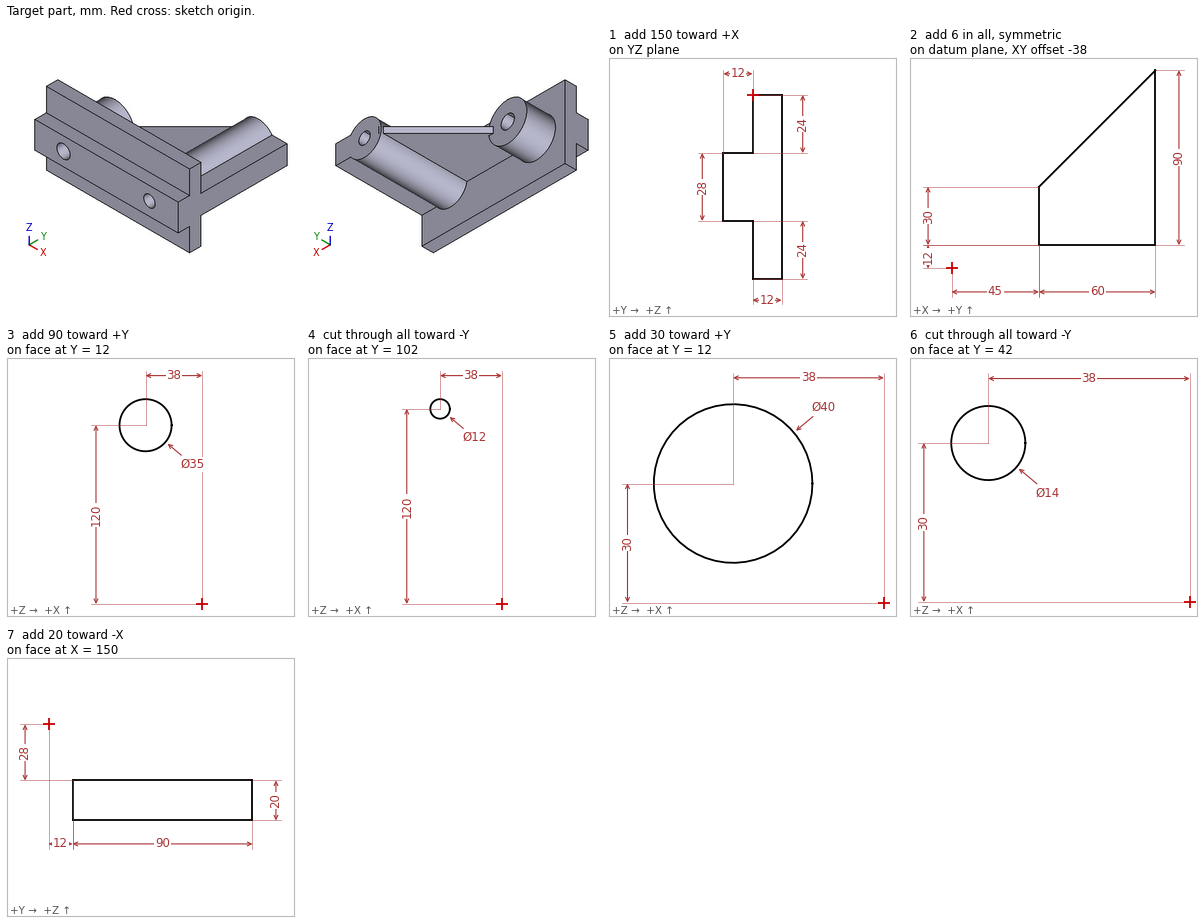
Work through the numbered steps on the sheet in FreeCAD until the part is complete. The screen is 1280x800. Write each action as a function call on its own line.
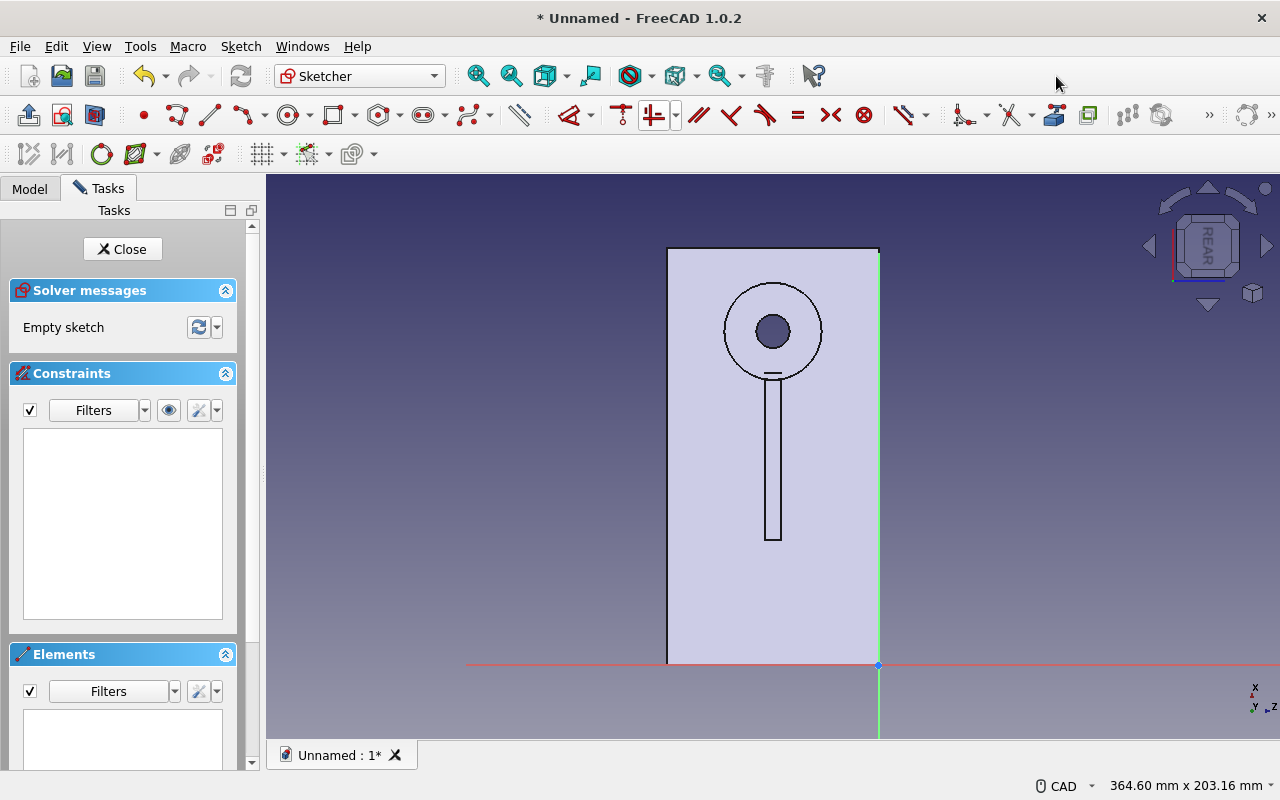
click(95, 116)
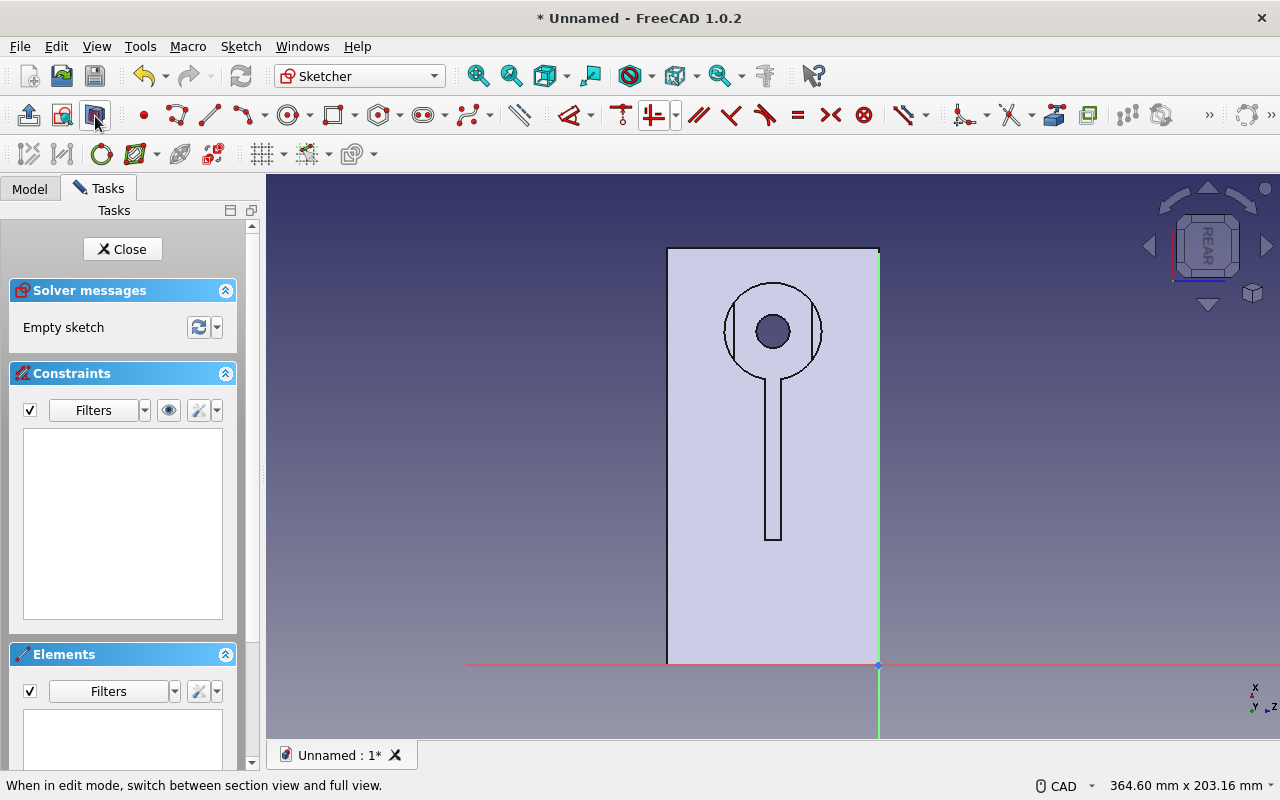
scroll(852, 676, up, 5)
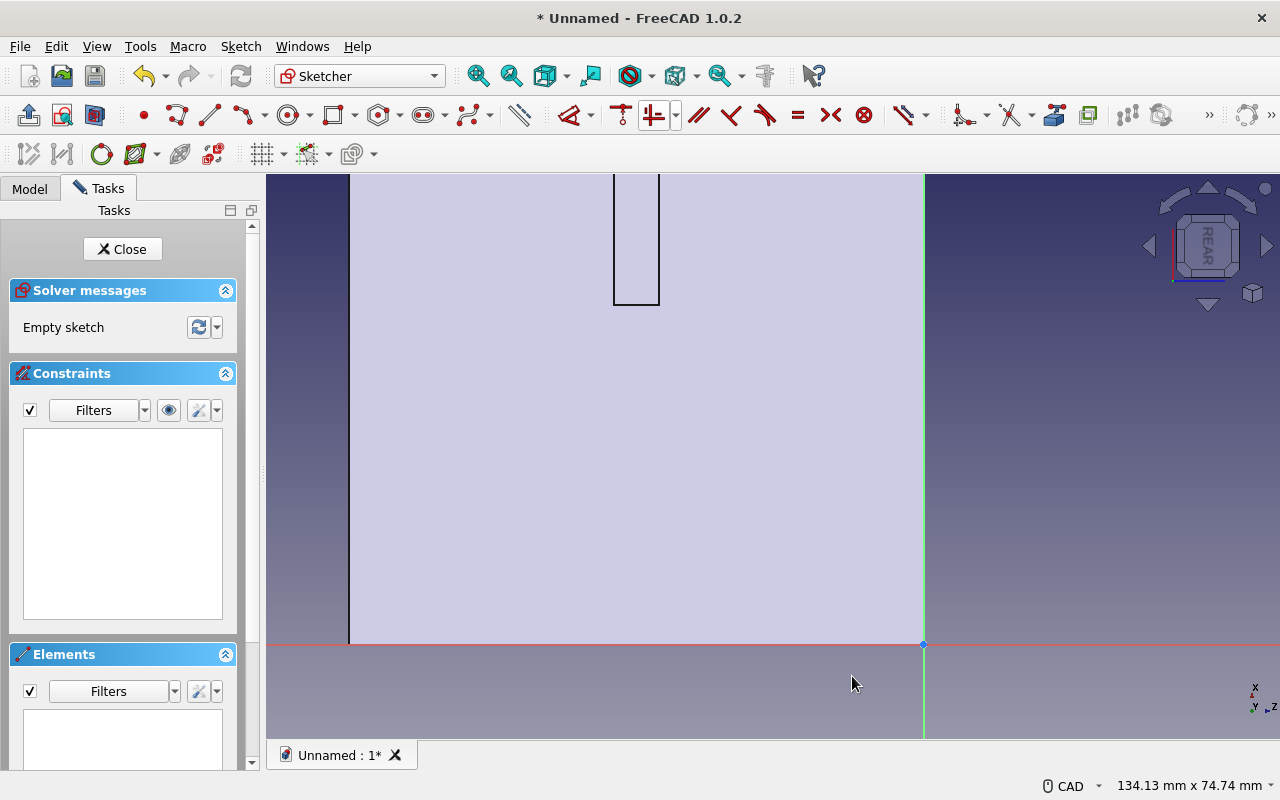
click(288, 116)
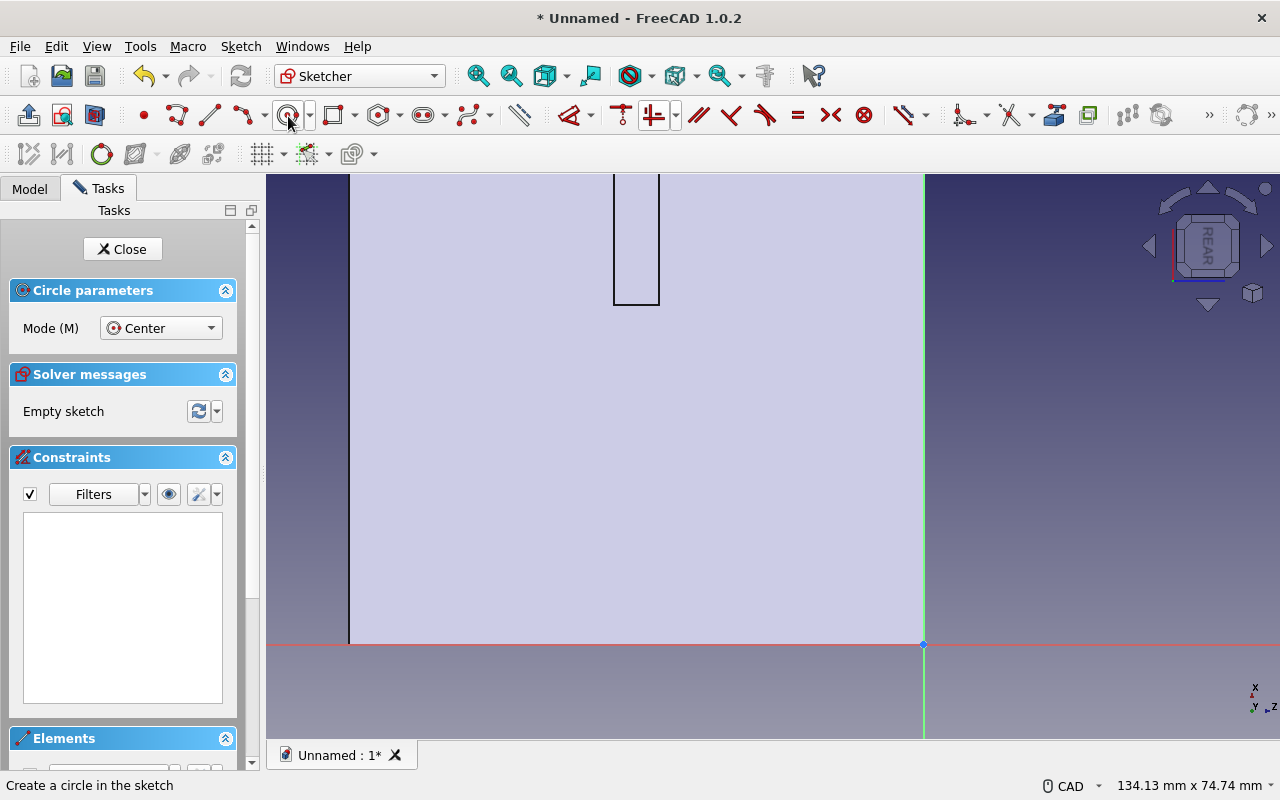
click(636, 418)
move(743, 311)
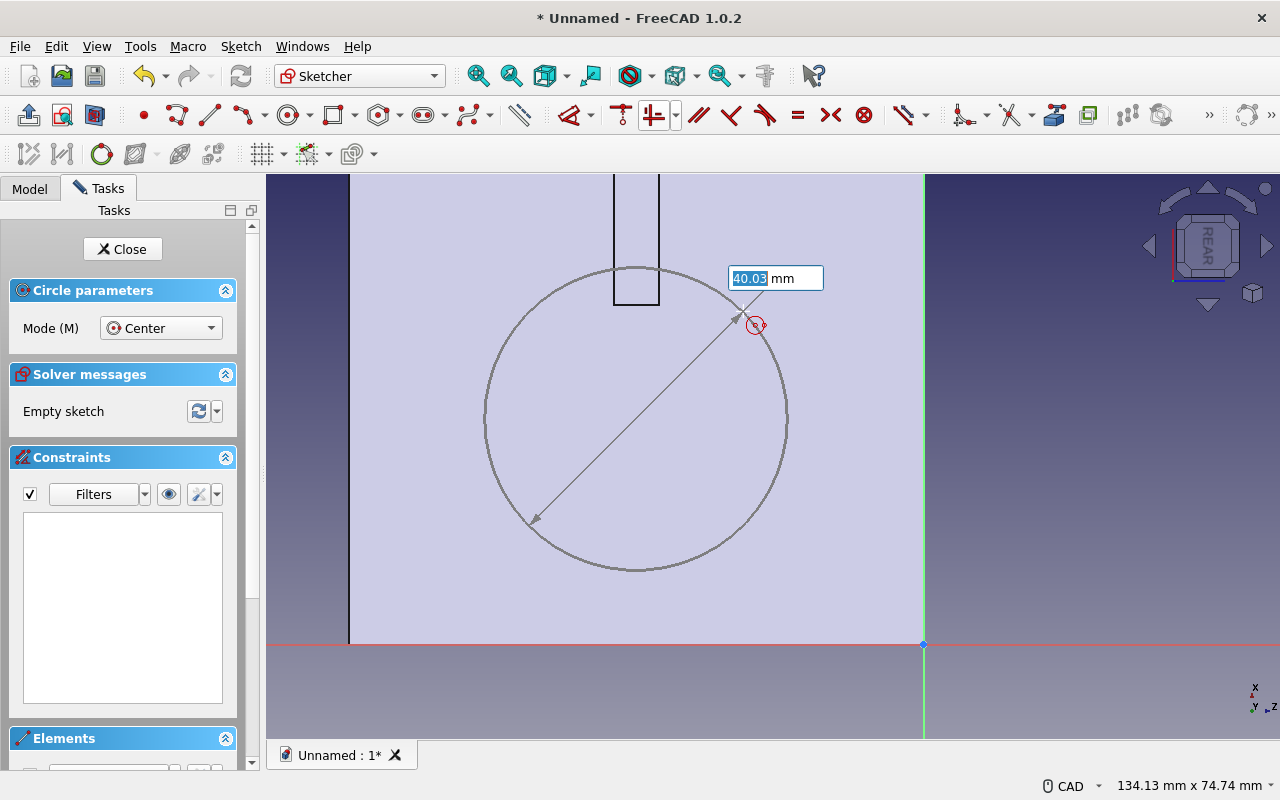
text(40)
key(Return)
key(Escape)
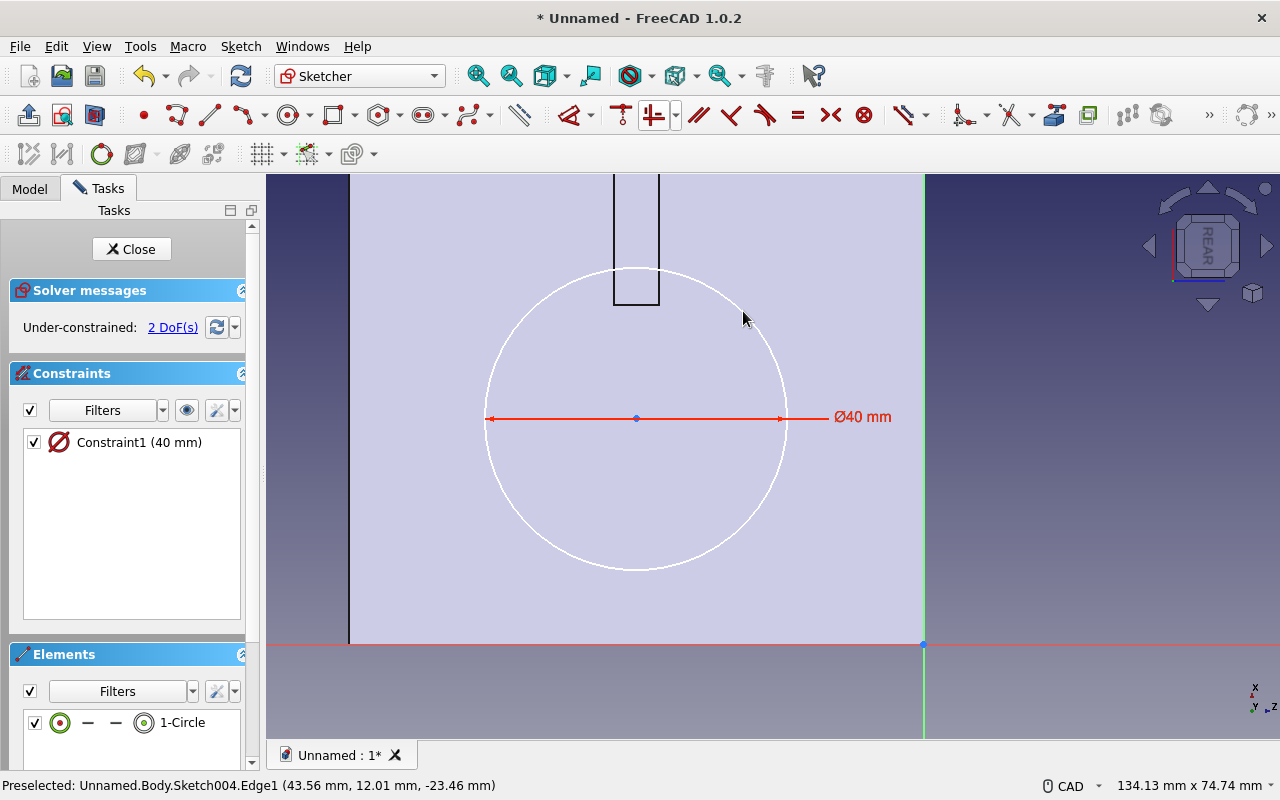
click(568, 116)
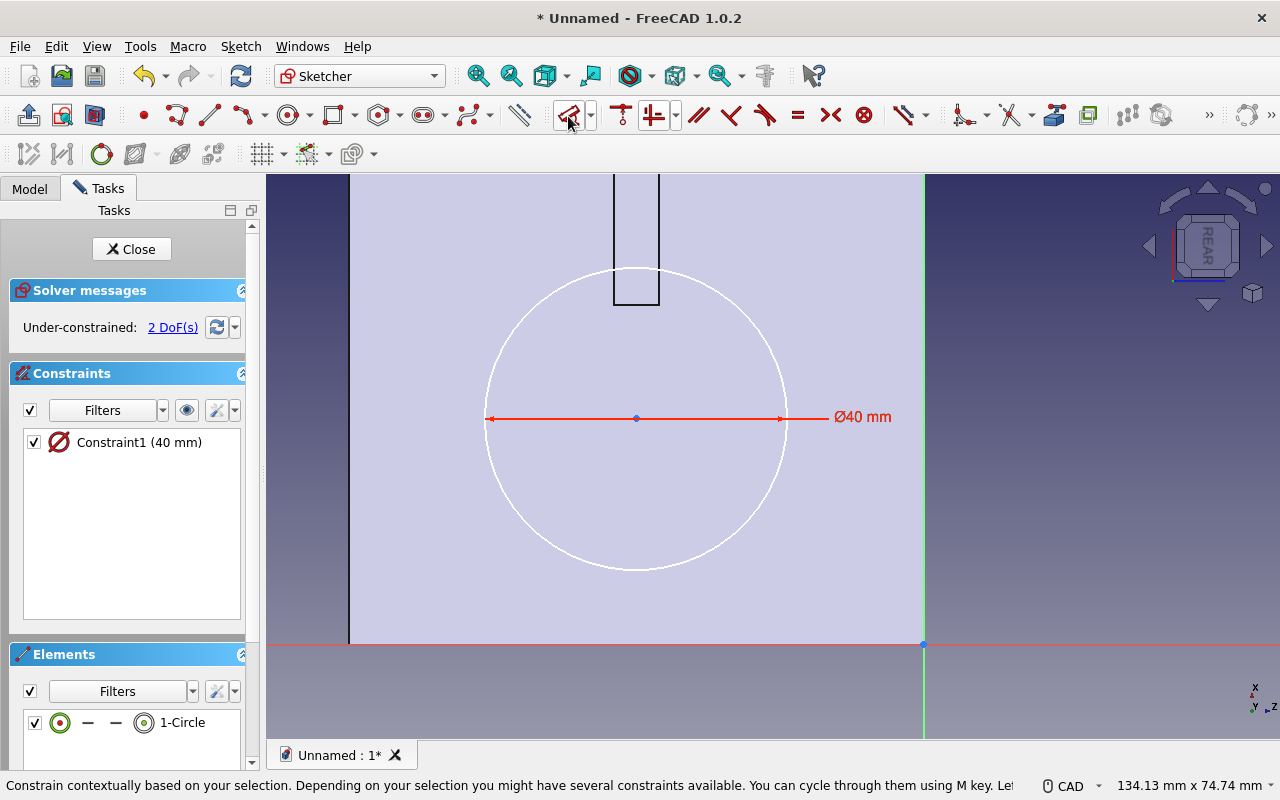
click(636, 419)
click(780, 679)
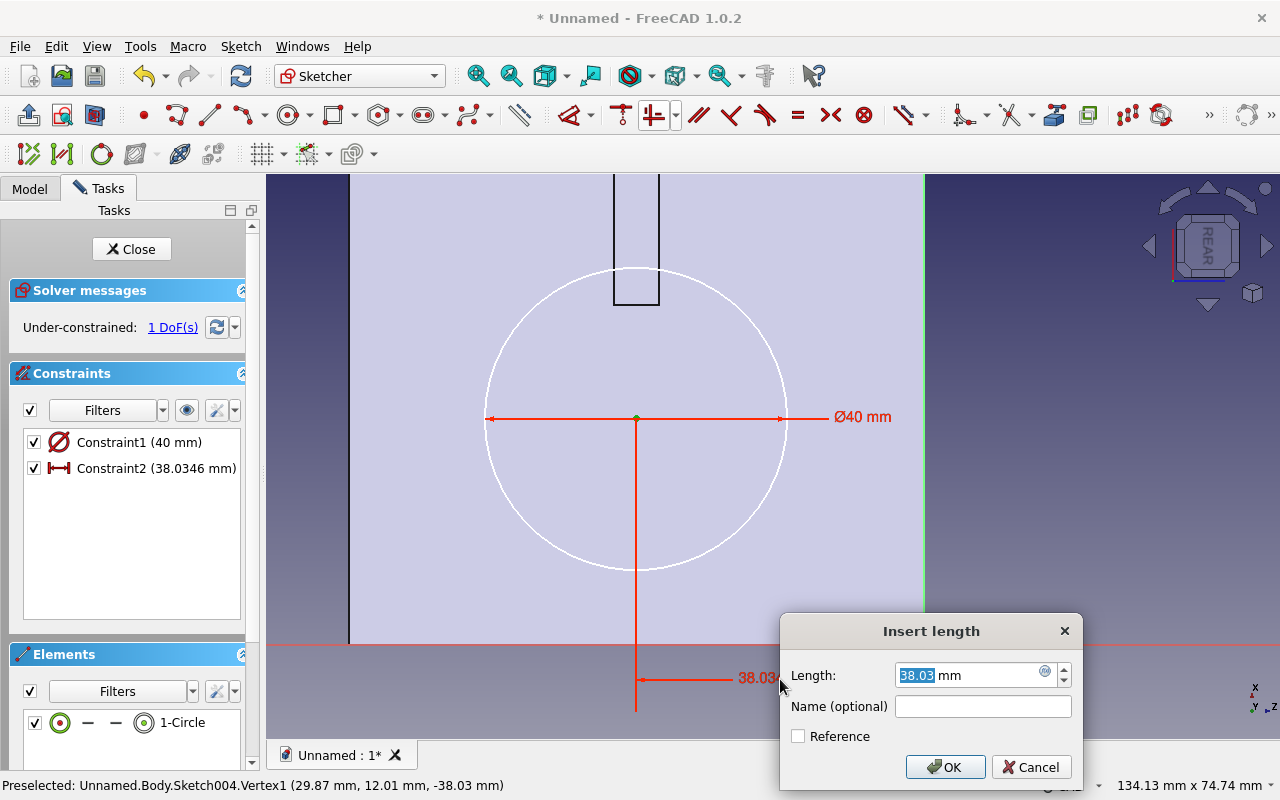
text(38)
key(Return)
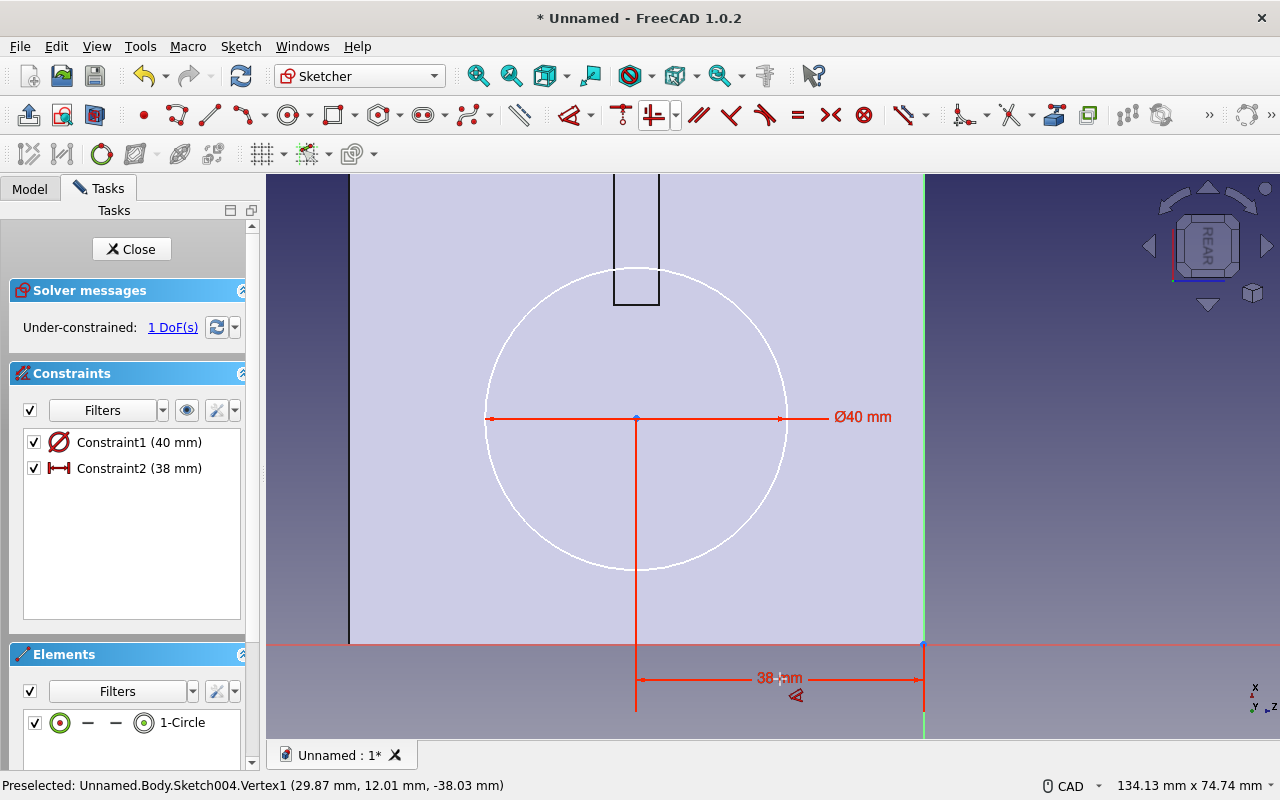
click(636, 419)
click(958, 532)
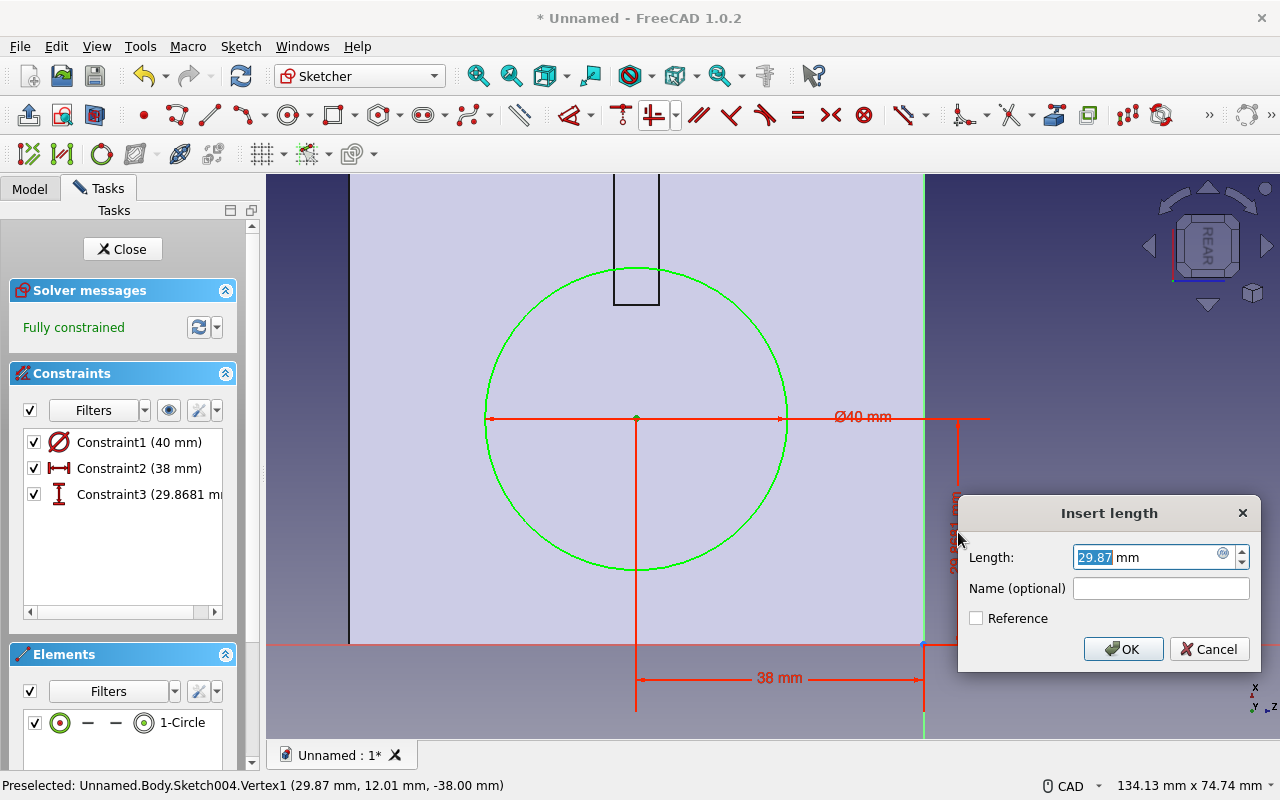
text(30)
key(Return)
key(Escape)